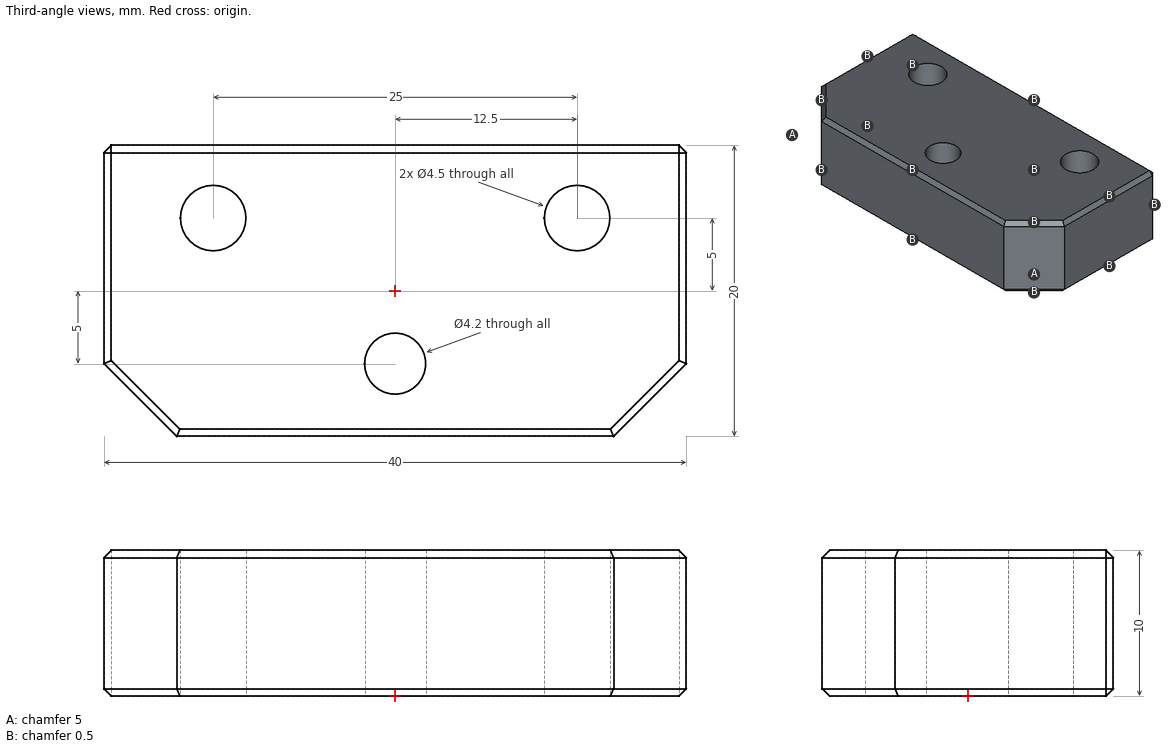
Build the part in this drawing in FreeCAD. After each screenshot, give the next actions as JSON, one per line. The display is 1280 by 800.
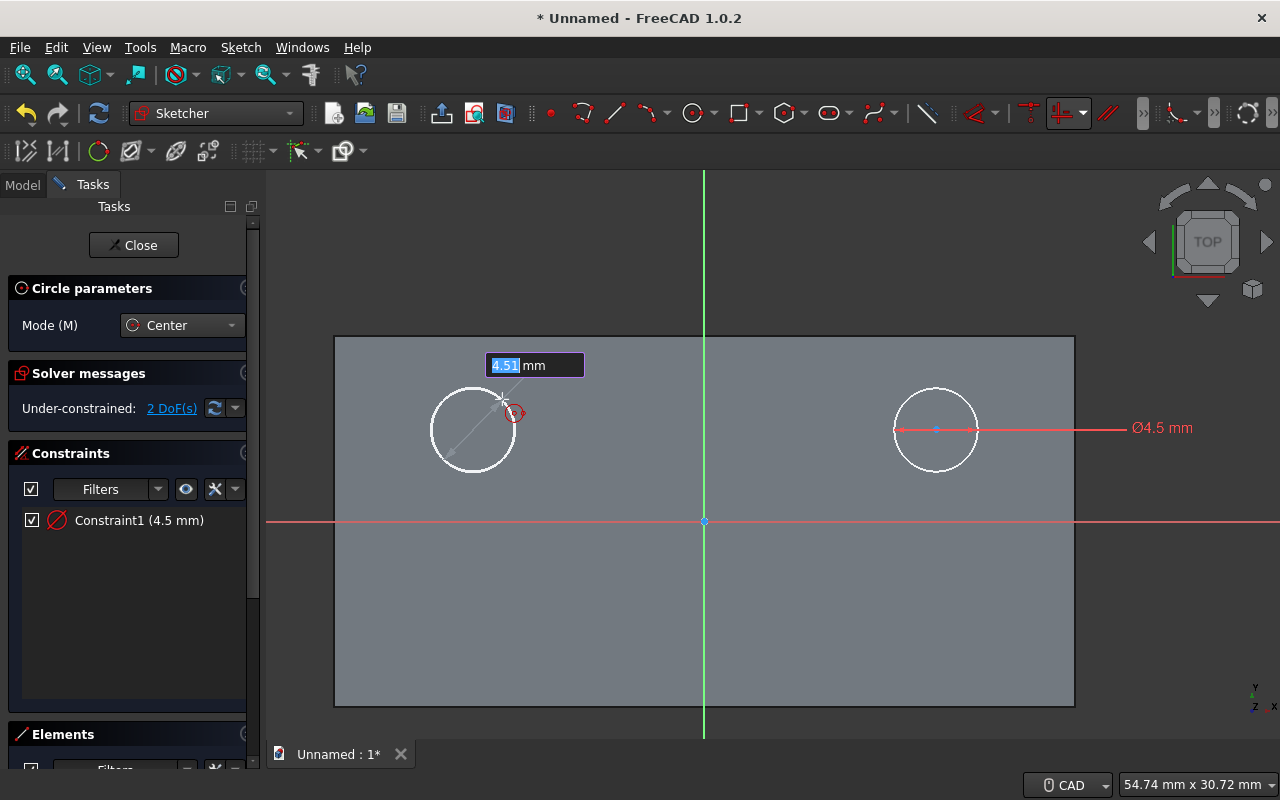
{"action": "type", "text": "4.5"}
{"action": "key", "text": "Return"}
{"action": "key", "text": "Escape"}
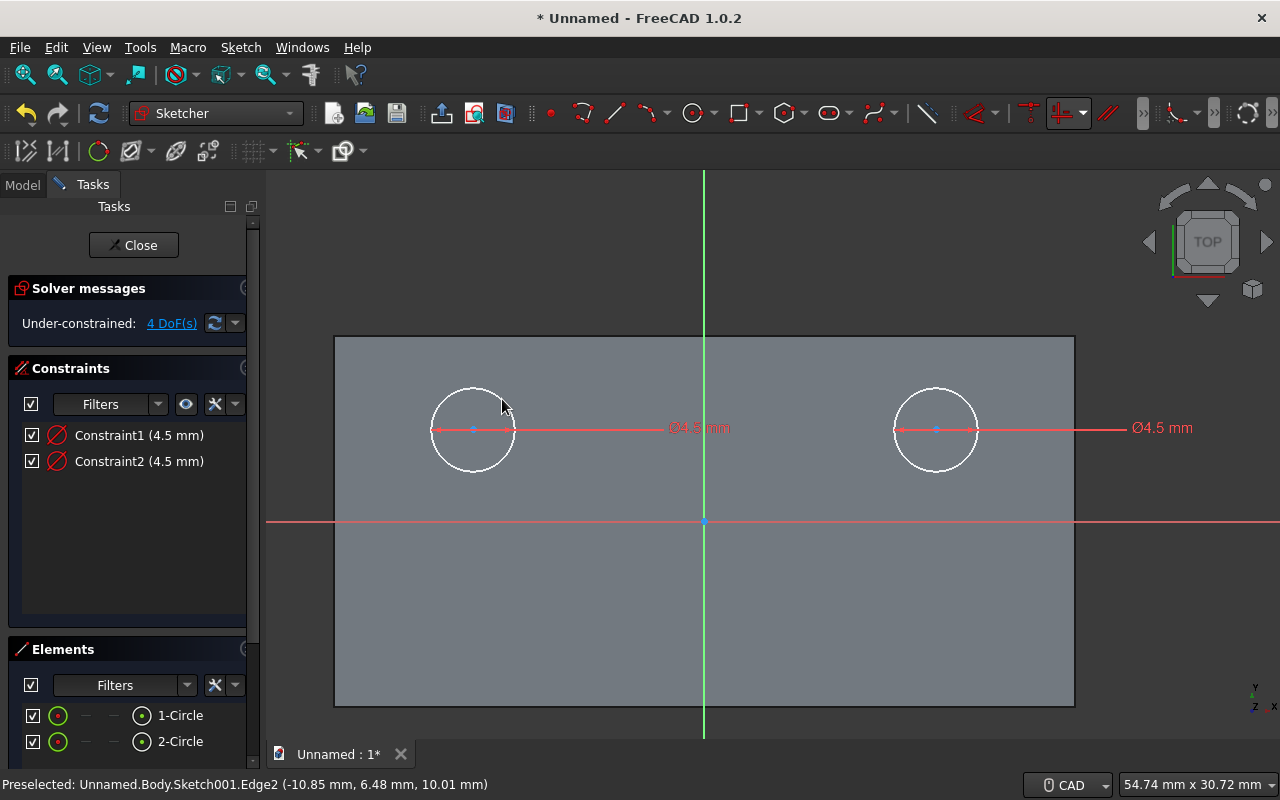
{"action": "left_click", "coordinate": [936, 430]}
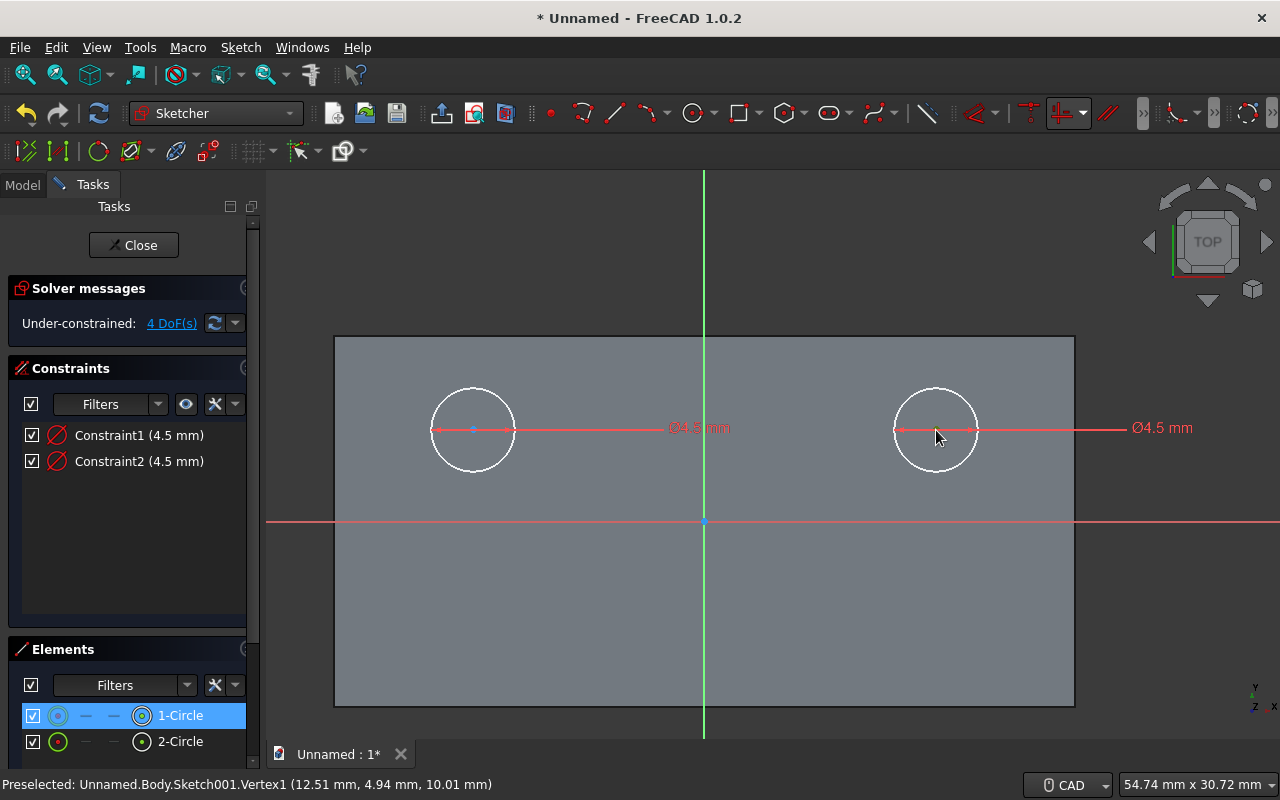
{"action": "left_click", "coordinate": [473, 430]}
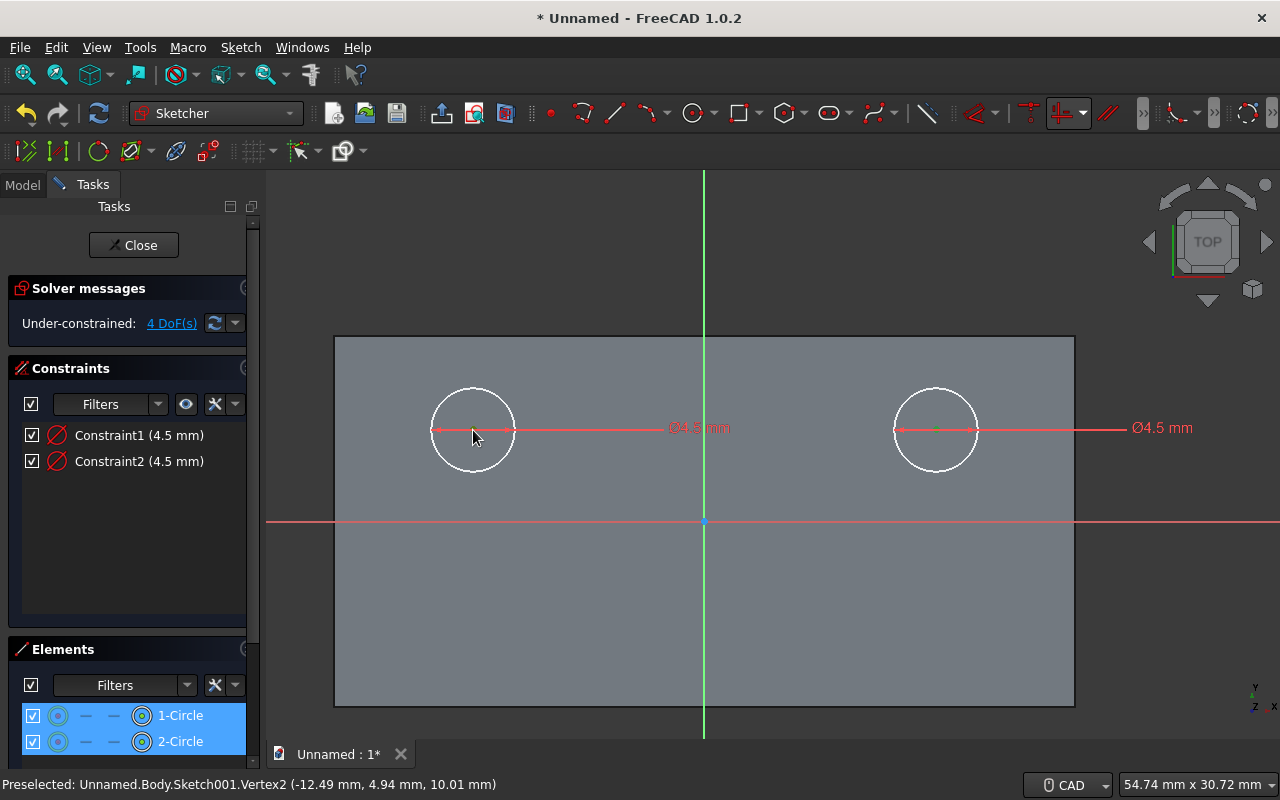
{"action": "left_click", "coordinate": [1086, 114]}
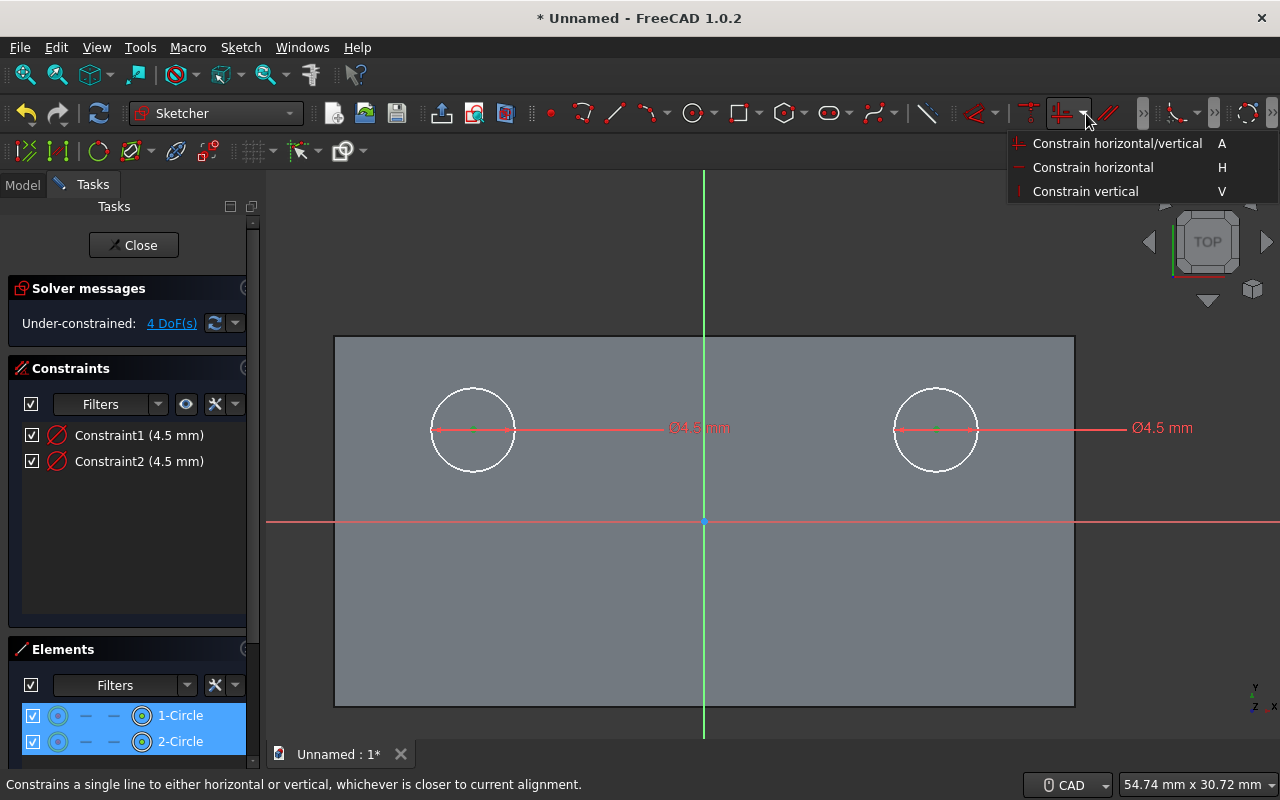
{"action": "left_click", "coordinate": [1143, 167]}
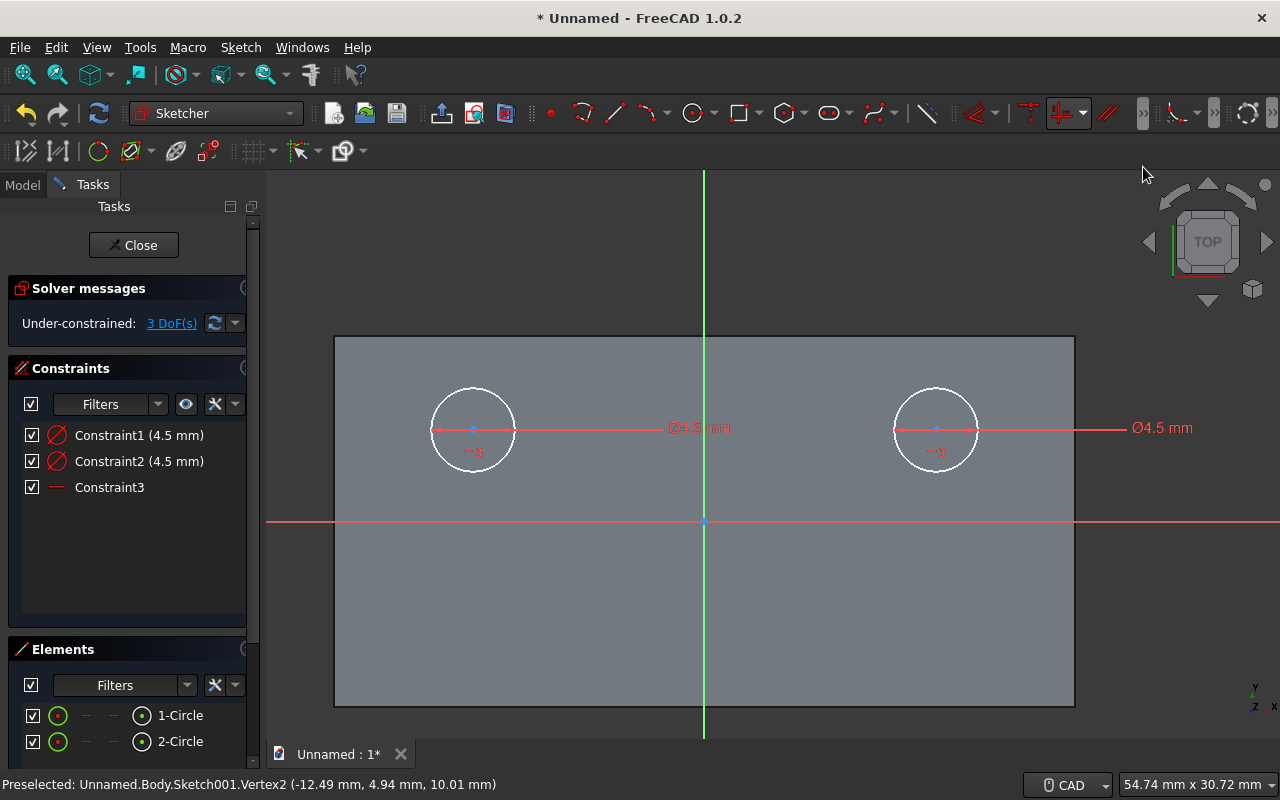
{"action": "left_click", "coordinate": [974, 114]}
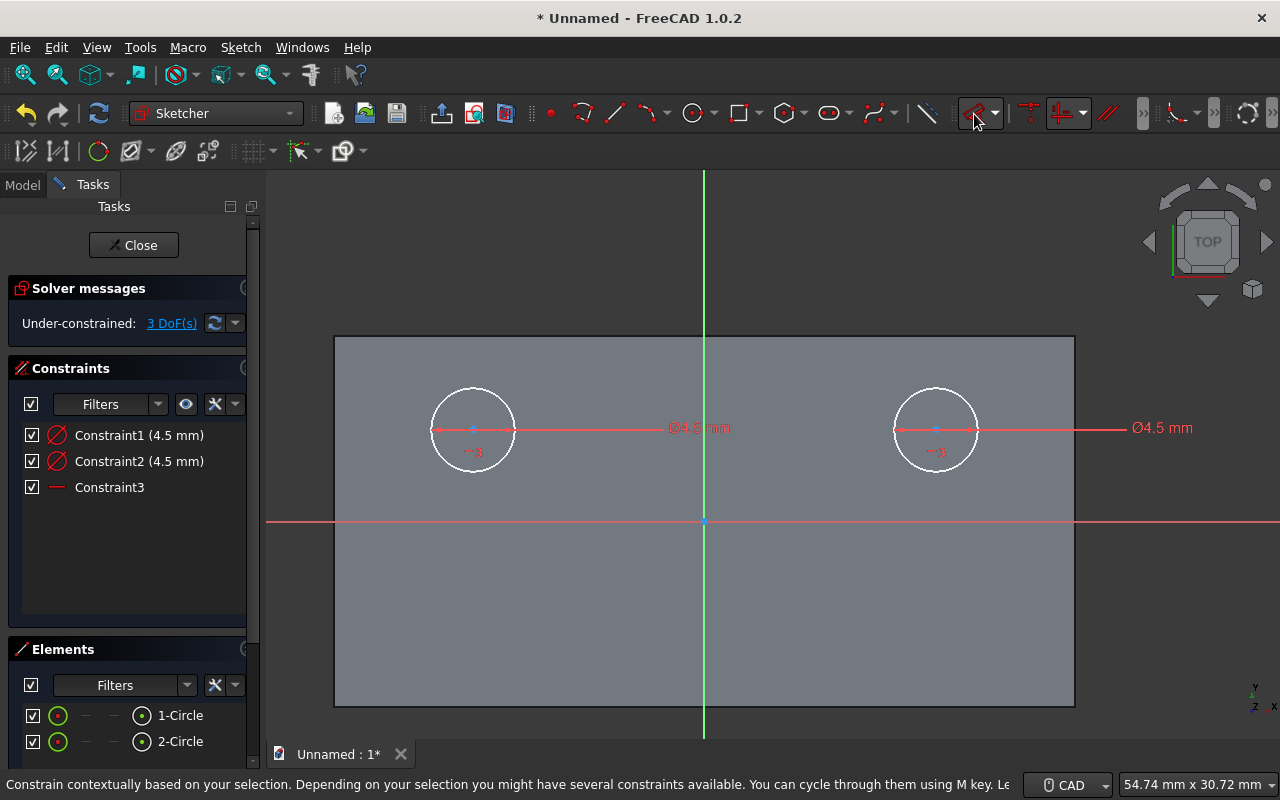
{"action": "left_click", "coordinate": [936, 430]}
{"action": "left_click", "coordinate": [970, 476]}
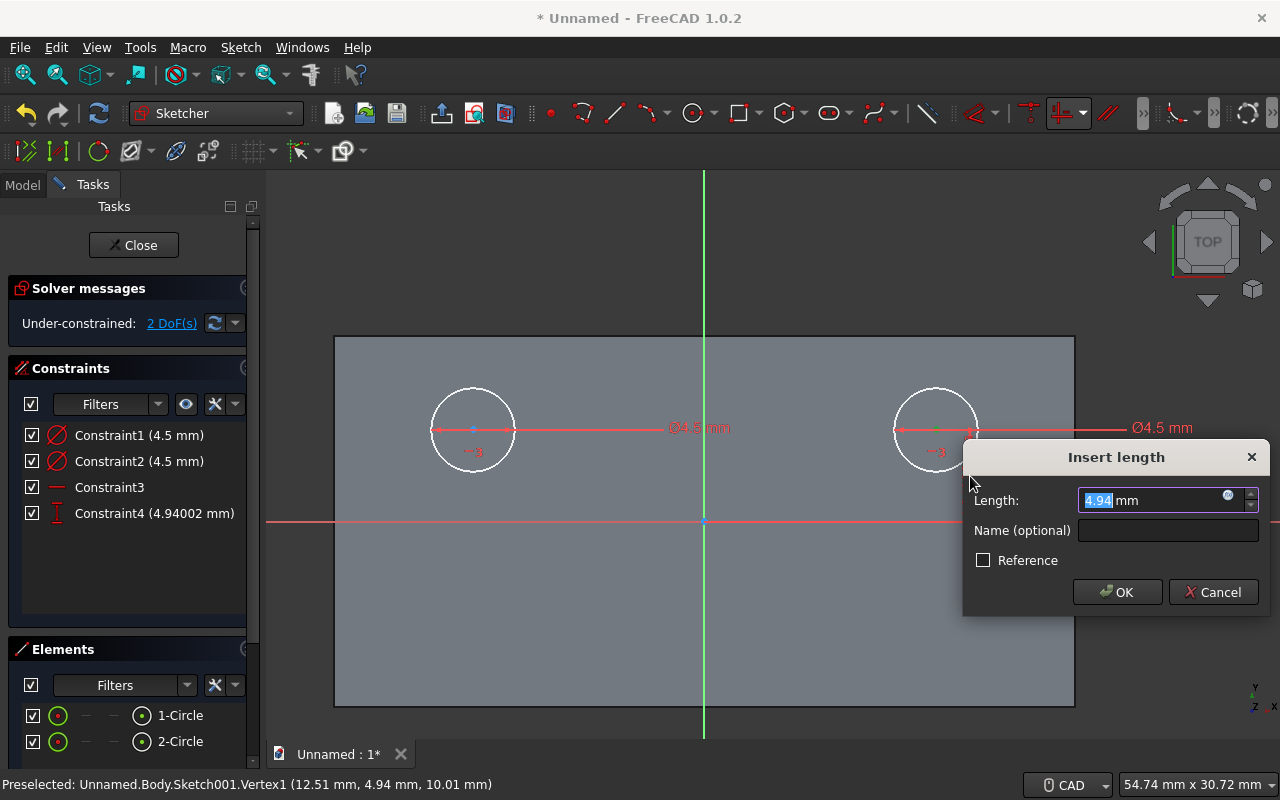
{"action": "type", "text": "5"}
{"action": "key", "text": "Return"}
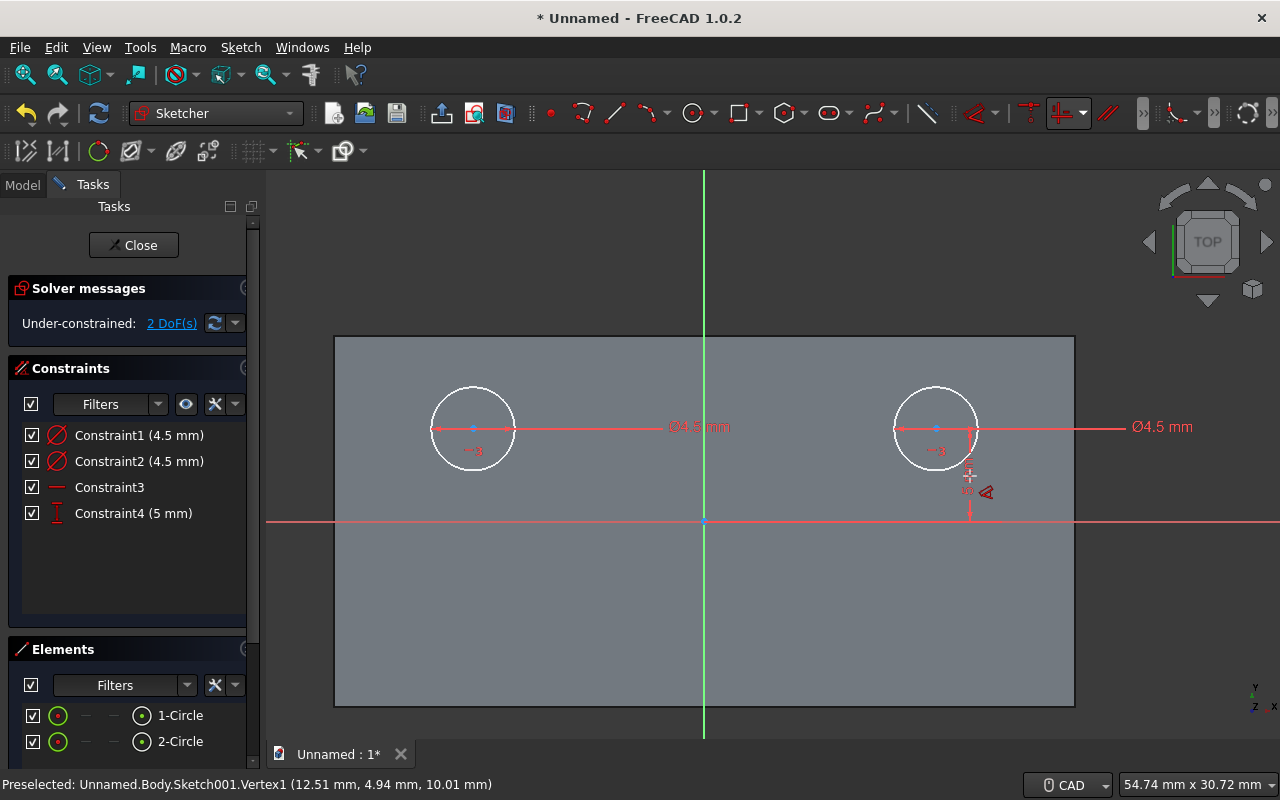
{"action": "left_click", "coordinate": [936, 429]}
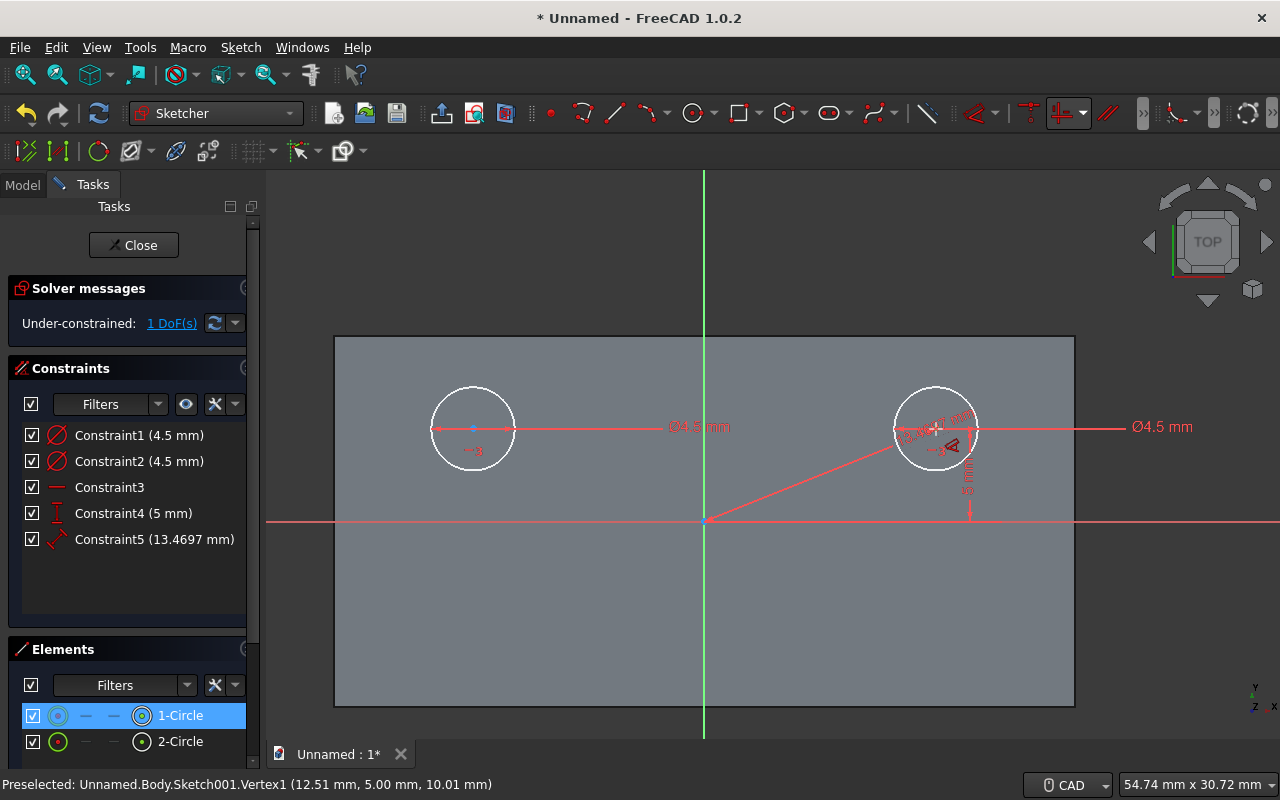
{"action": "left_click", "coordinate": [473, 429]}
{"action": "left_click", "coordinate": [598, 395]}